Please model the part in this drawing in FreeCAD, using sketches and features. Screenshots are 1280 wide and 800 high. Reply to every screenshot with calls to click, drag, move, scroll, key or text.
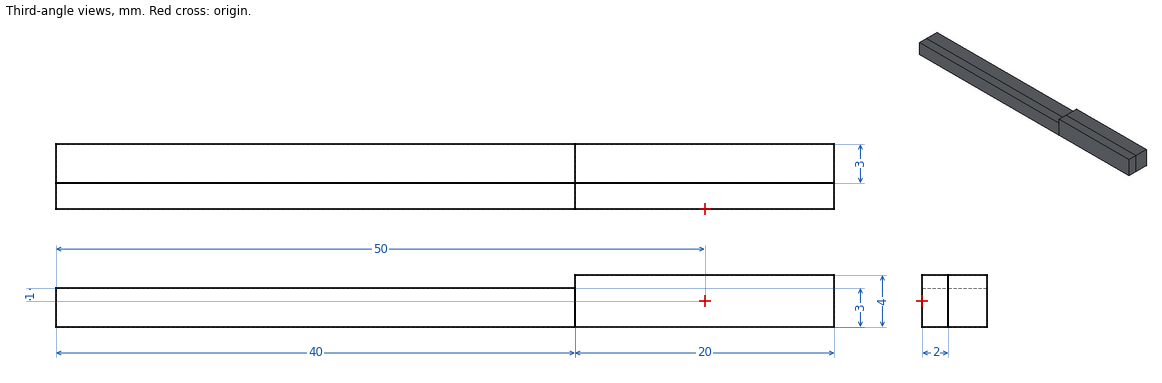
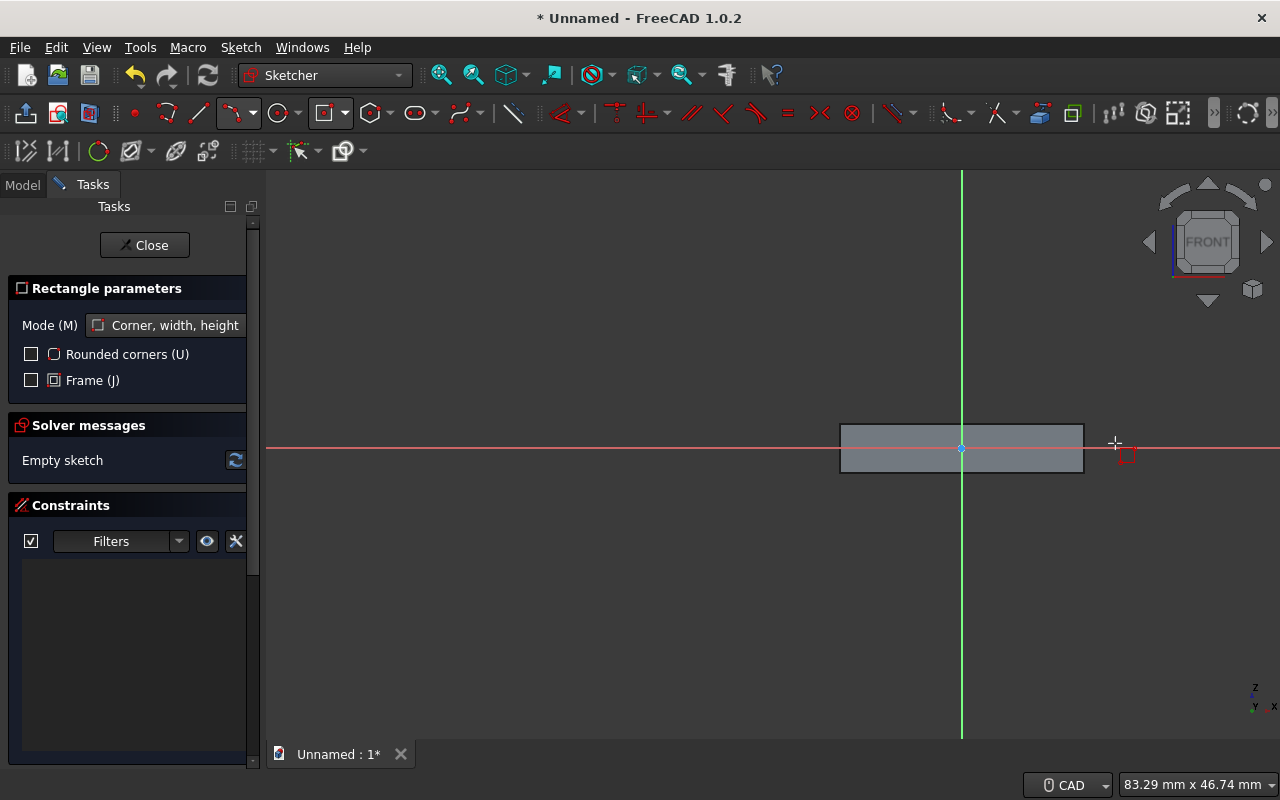
scroll(353, 436, up, 2)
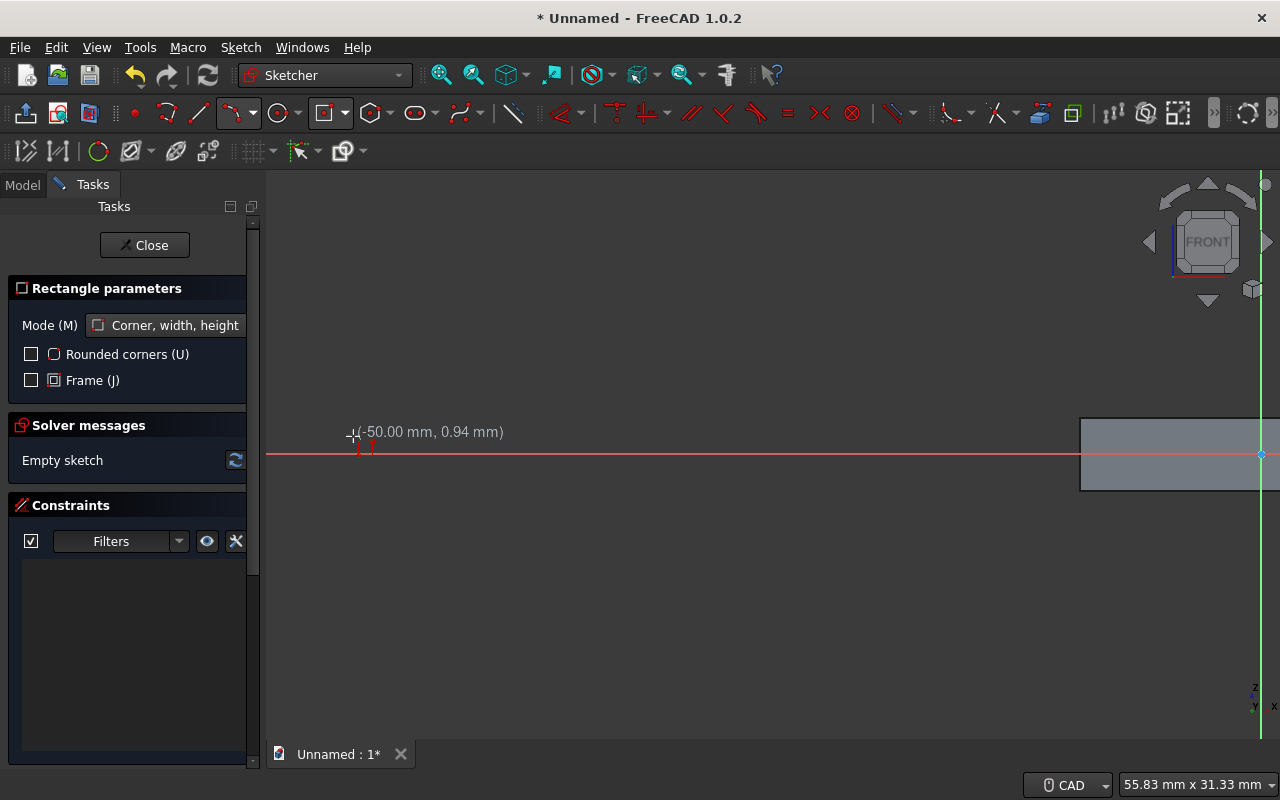
click(353, 436)
move(1080, 491)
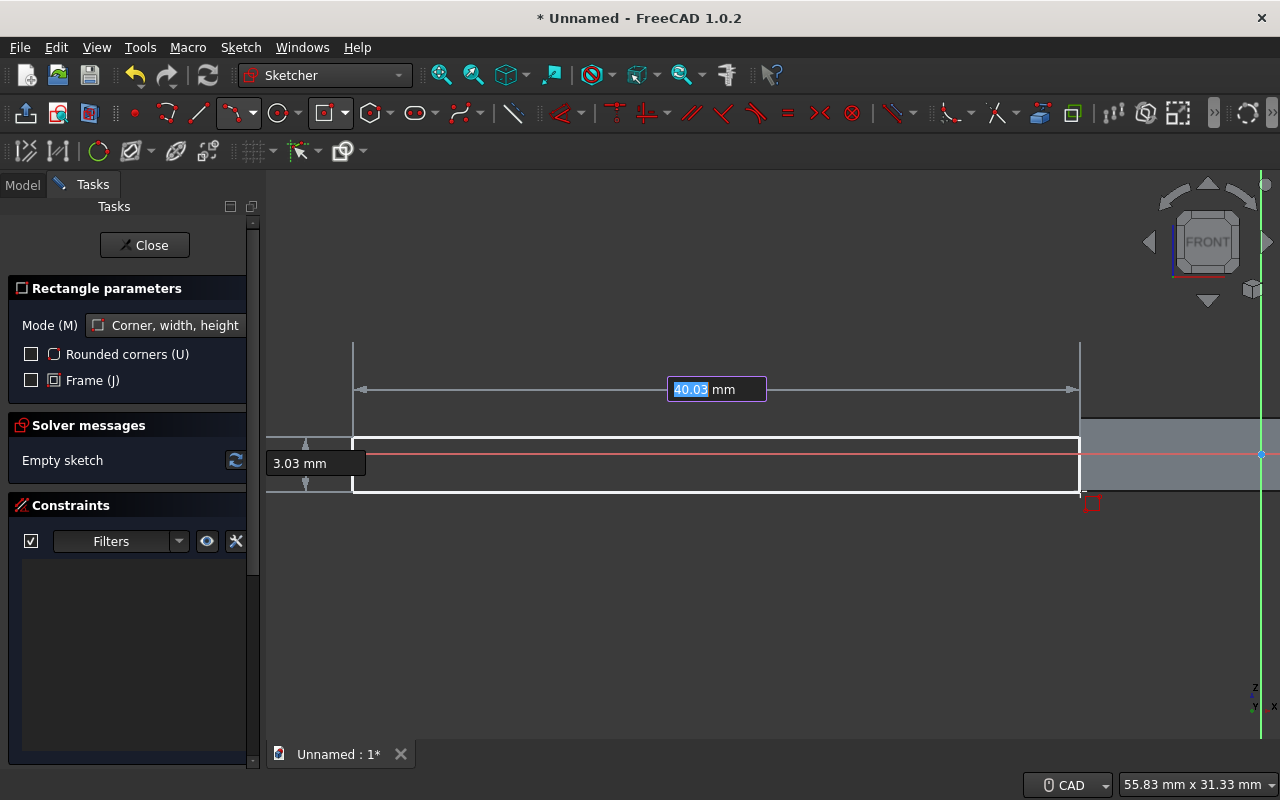
text(40)
key(Tab)
text(3)
key(Return)
key(Escape)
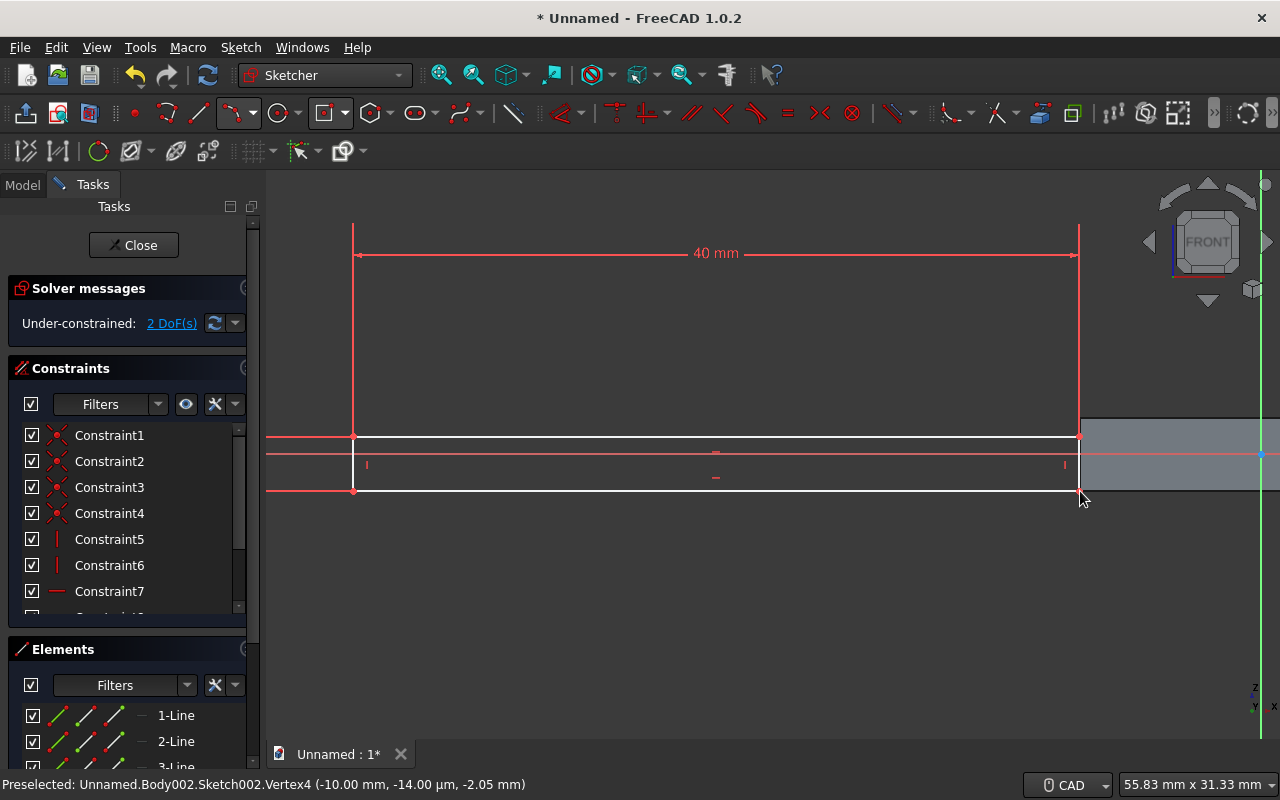
key(d)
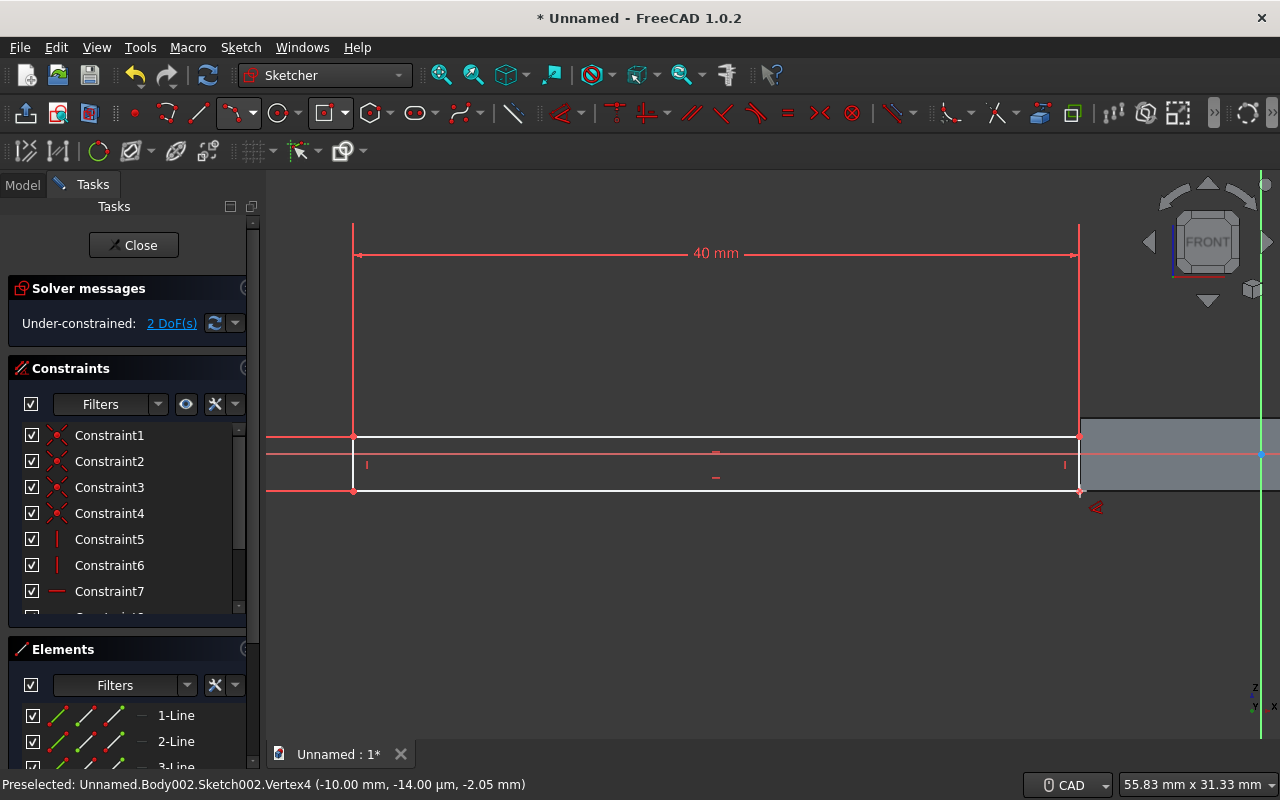
scroll(353, 437, up, 4)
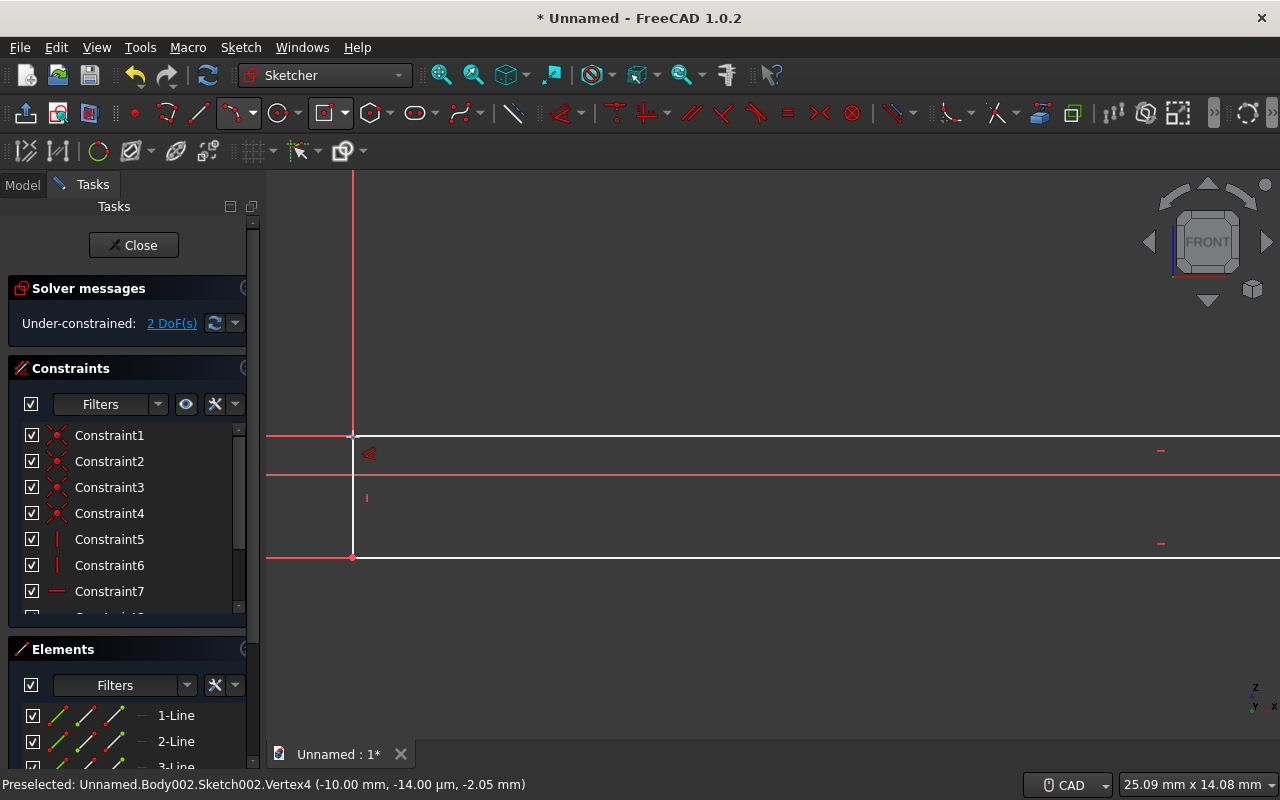
click(353, 436)
click(319, 456)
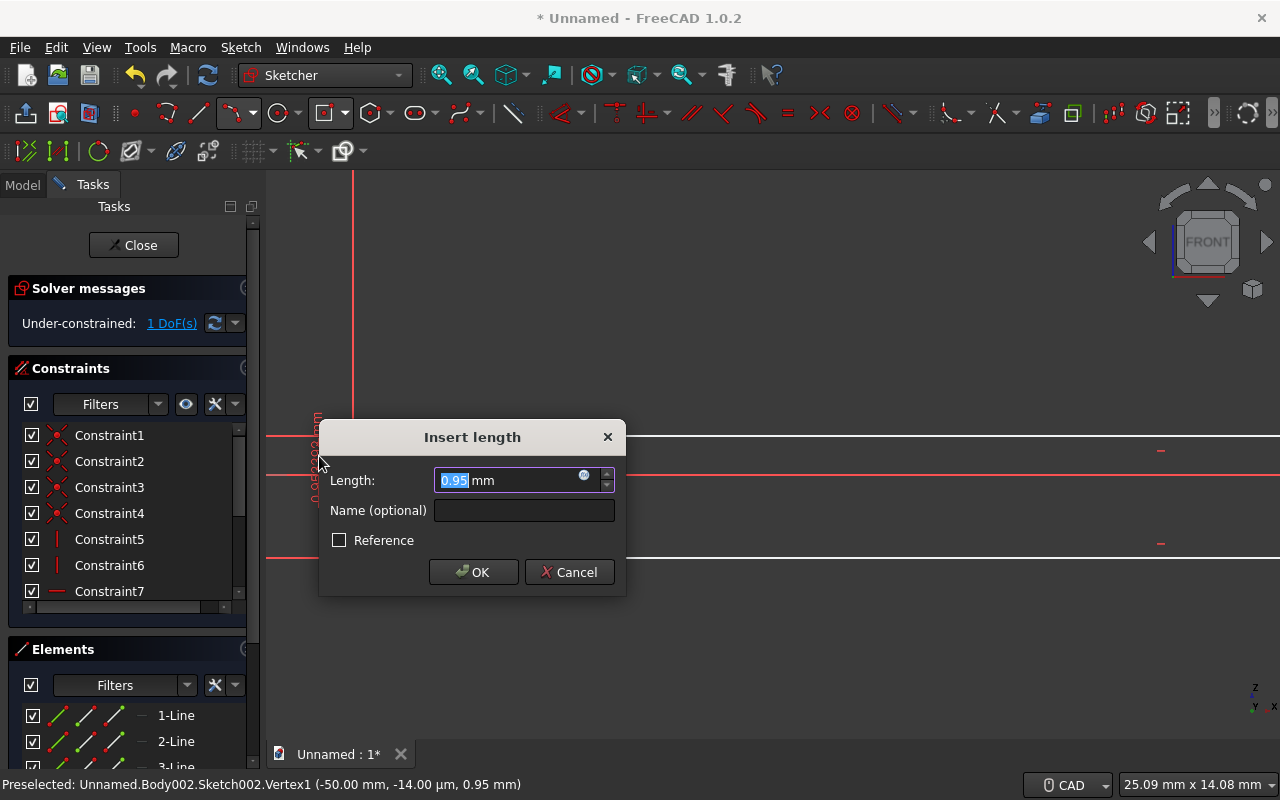
text(1)
key(Return)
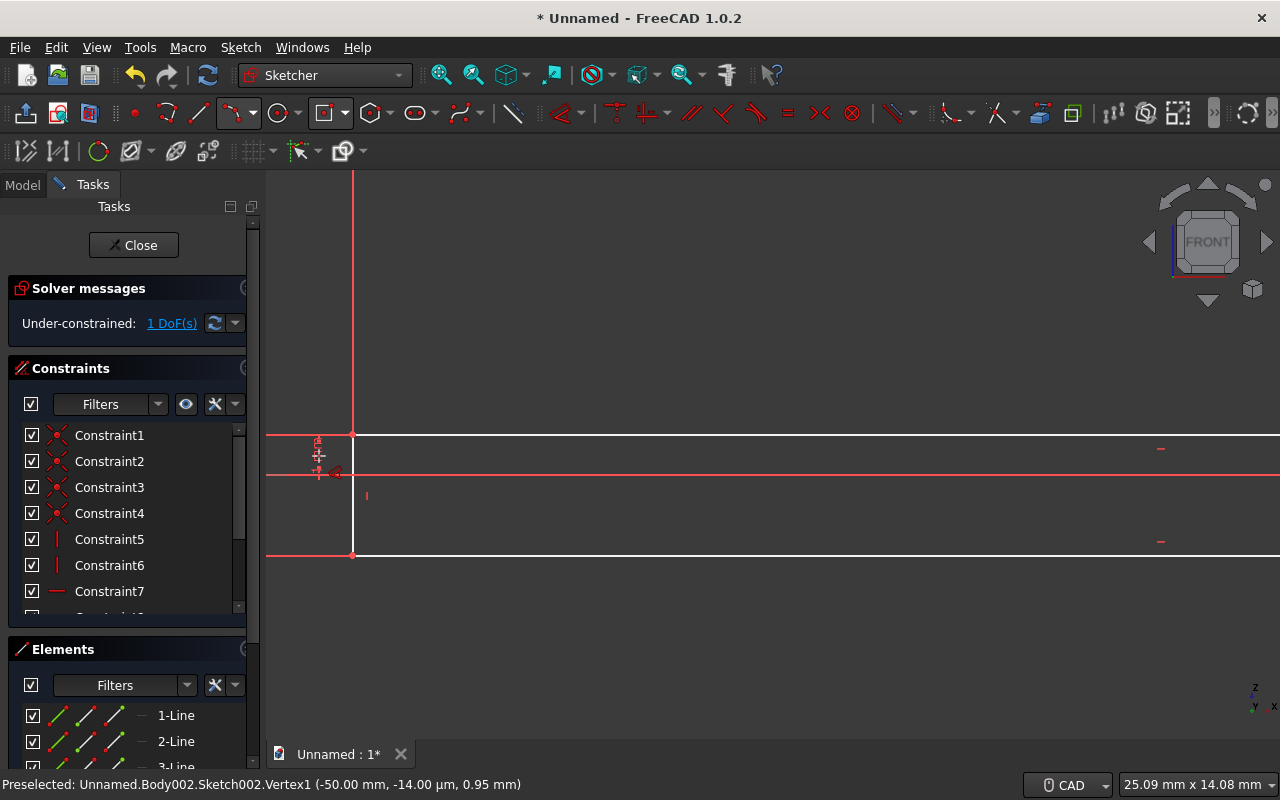
click(353, 435)
click(734, 401)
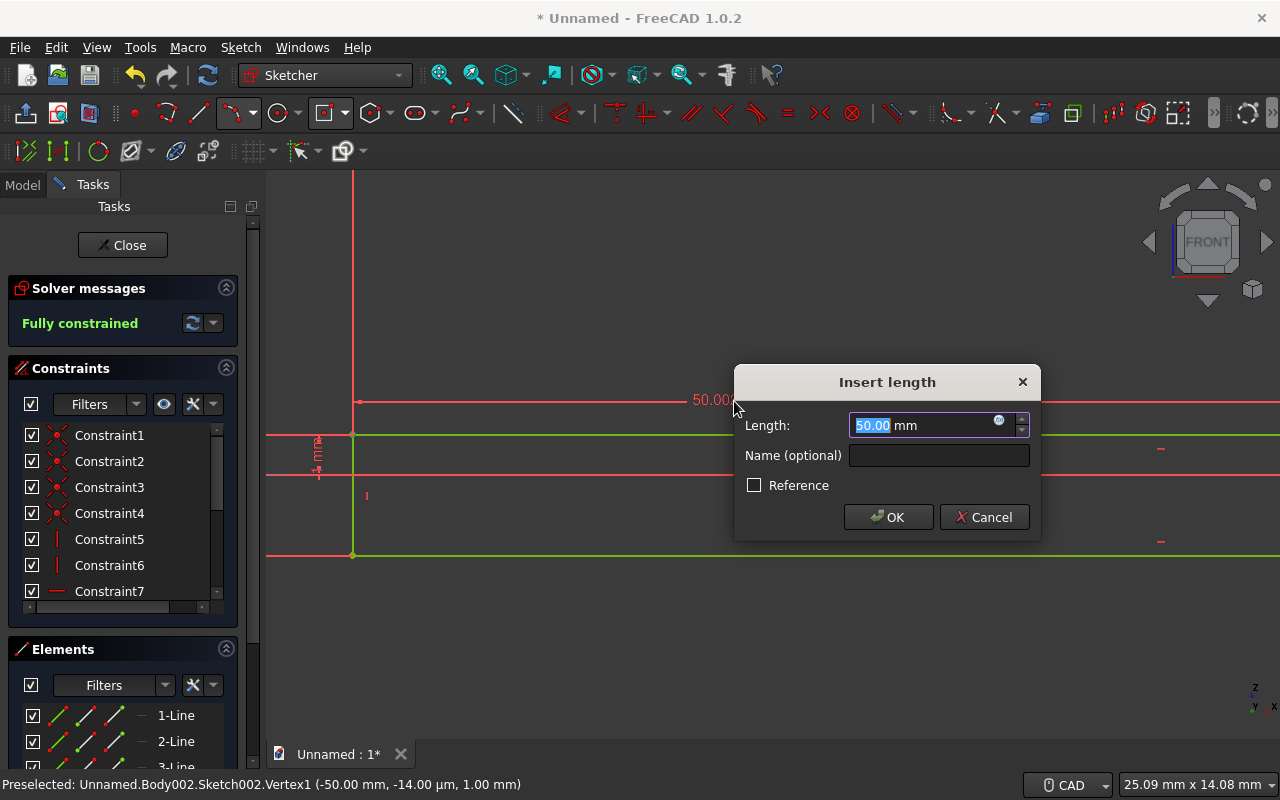
text(50)
key(Return)
key(Escape)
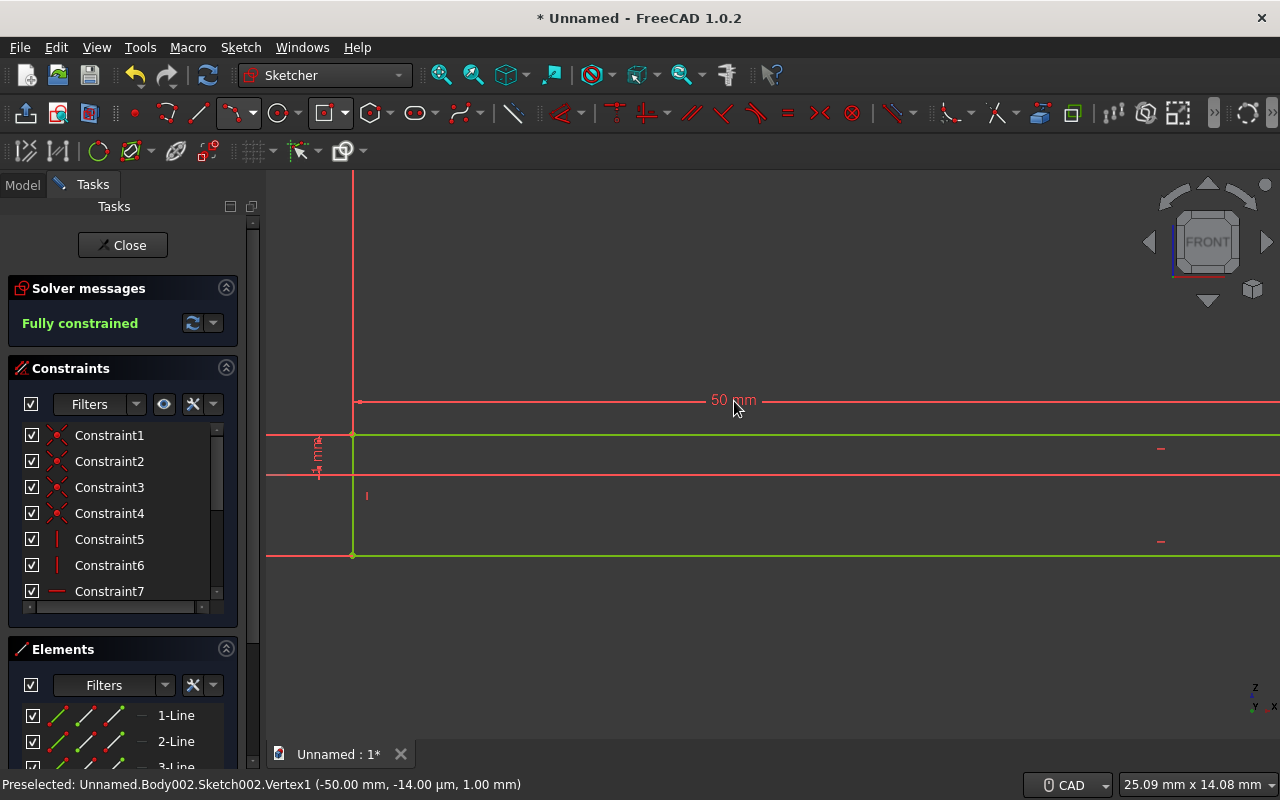
click(123, 245)